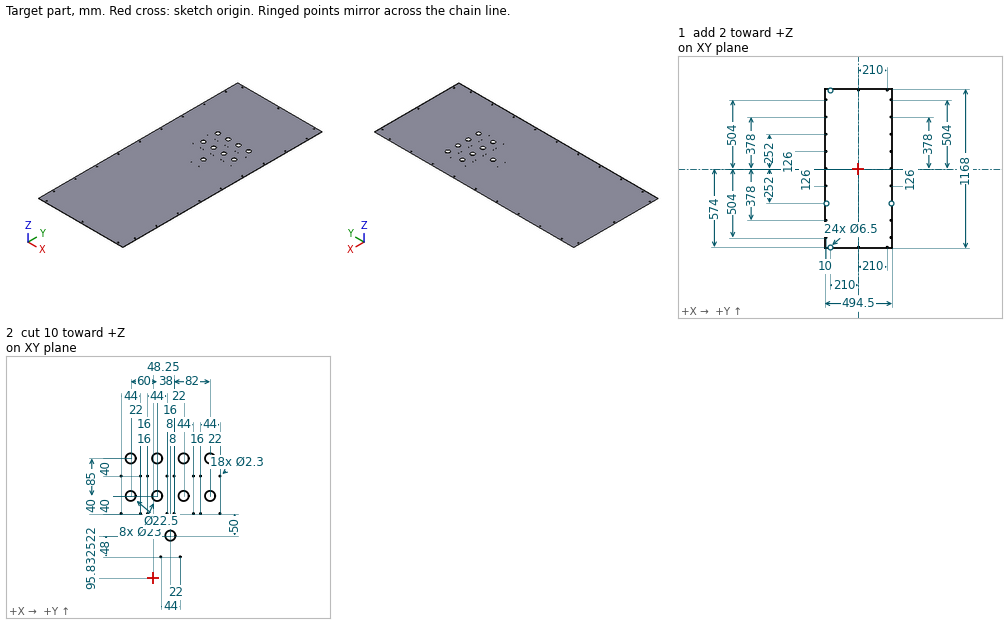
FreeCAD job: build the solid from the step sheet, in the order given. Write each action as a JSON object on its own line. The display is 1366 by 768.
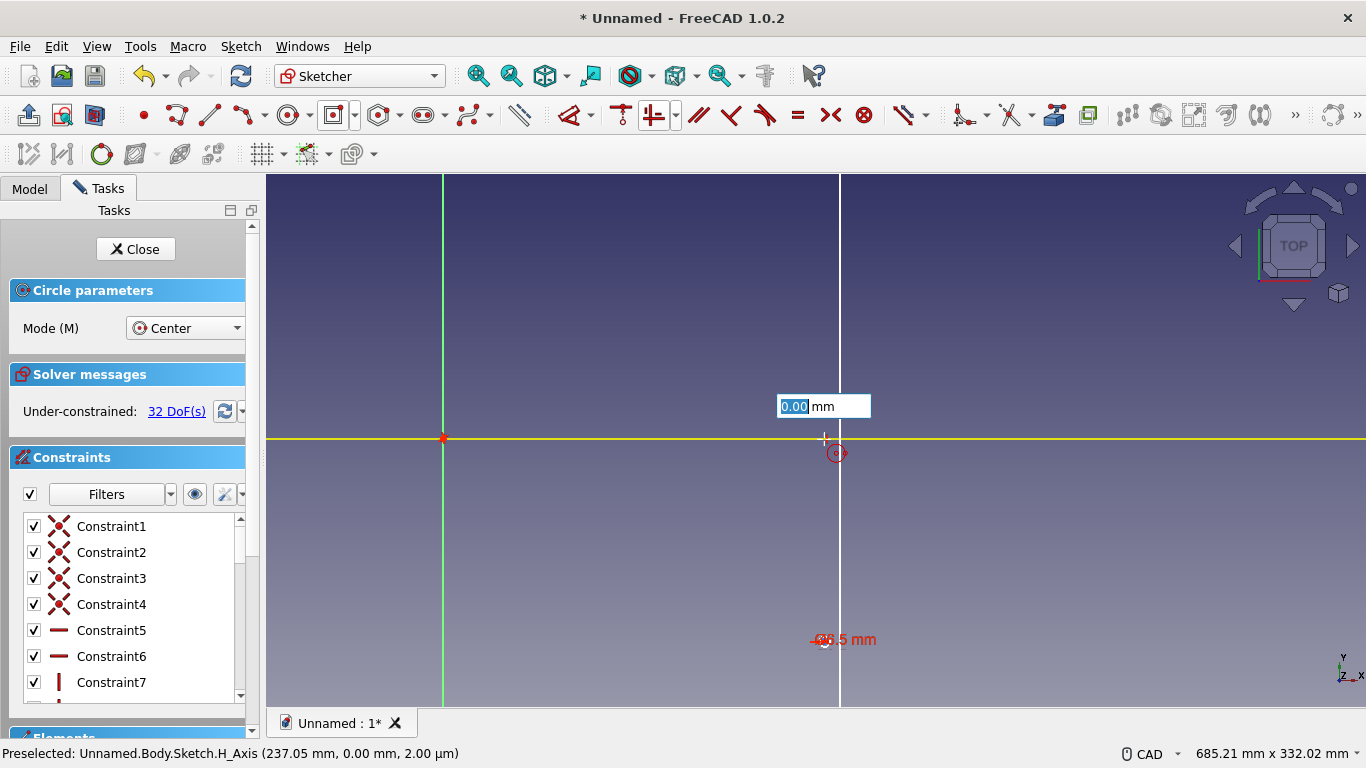
{"action": "scroll", "coordinate": [823, 443], "scroll_direction": "up", "scroll_amount": 6}
{"action": "mouse_move", "coordinate": [820, 443]}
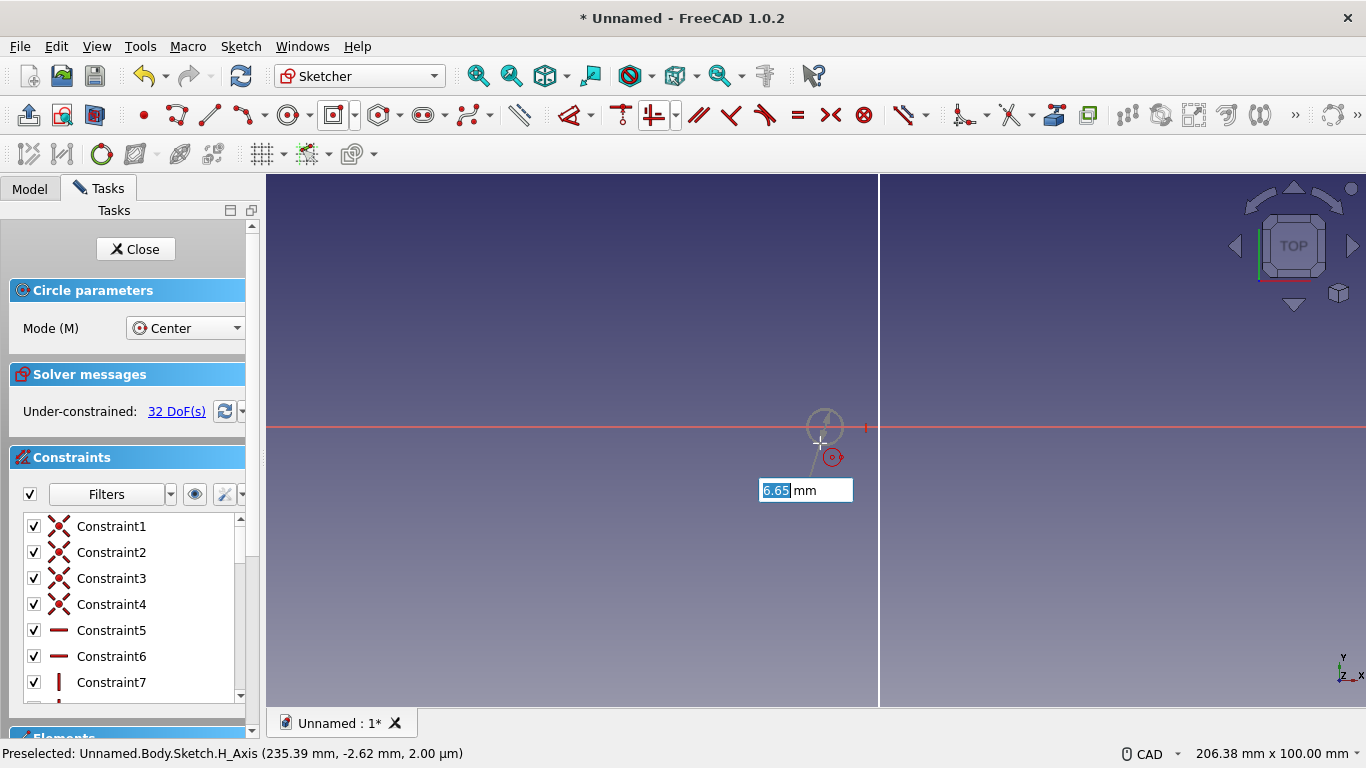
{"action": "type", "text": "6.5"}
{"action": "key", "text": "Return"}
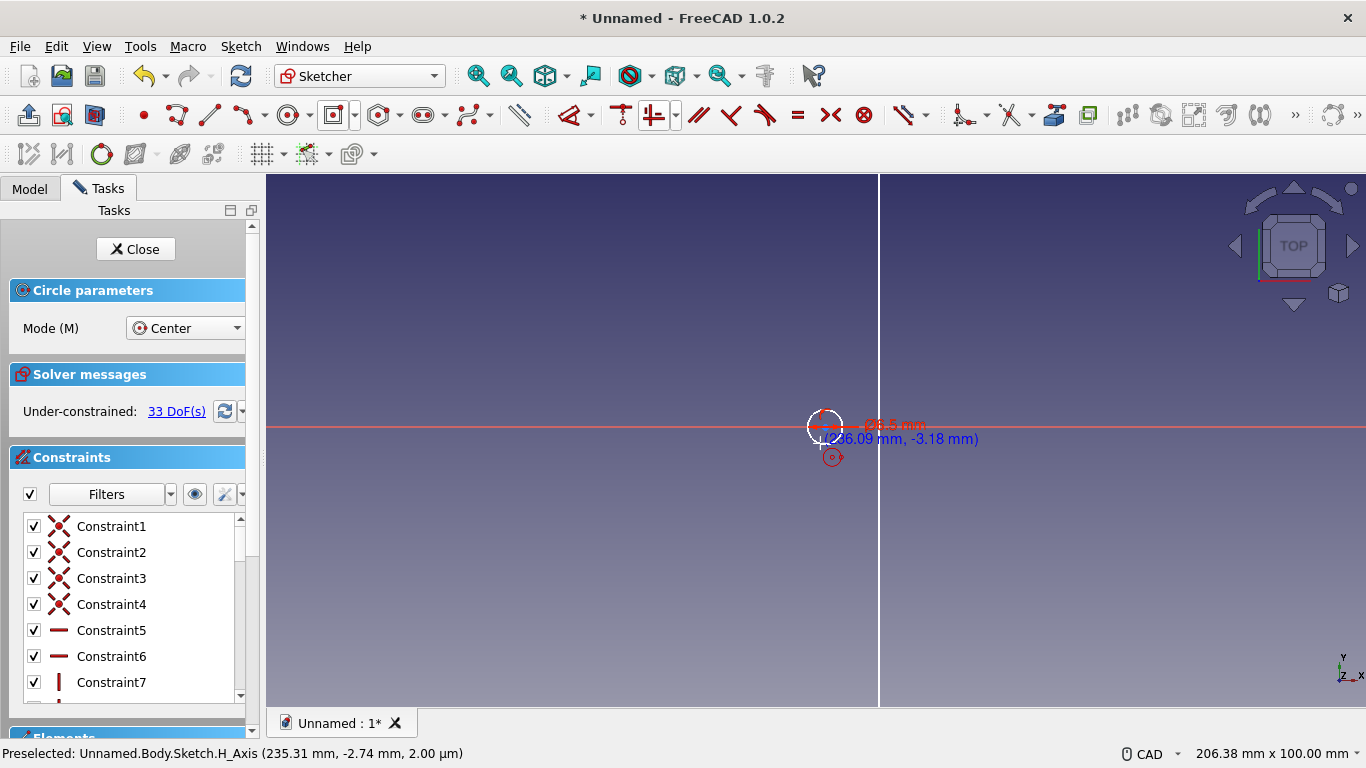
{"action": "scroll", "coordinate": [810, 441], "scroll_direction": "down", "scroll_amount": 15}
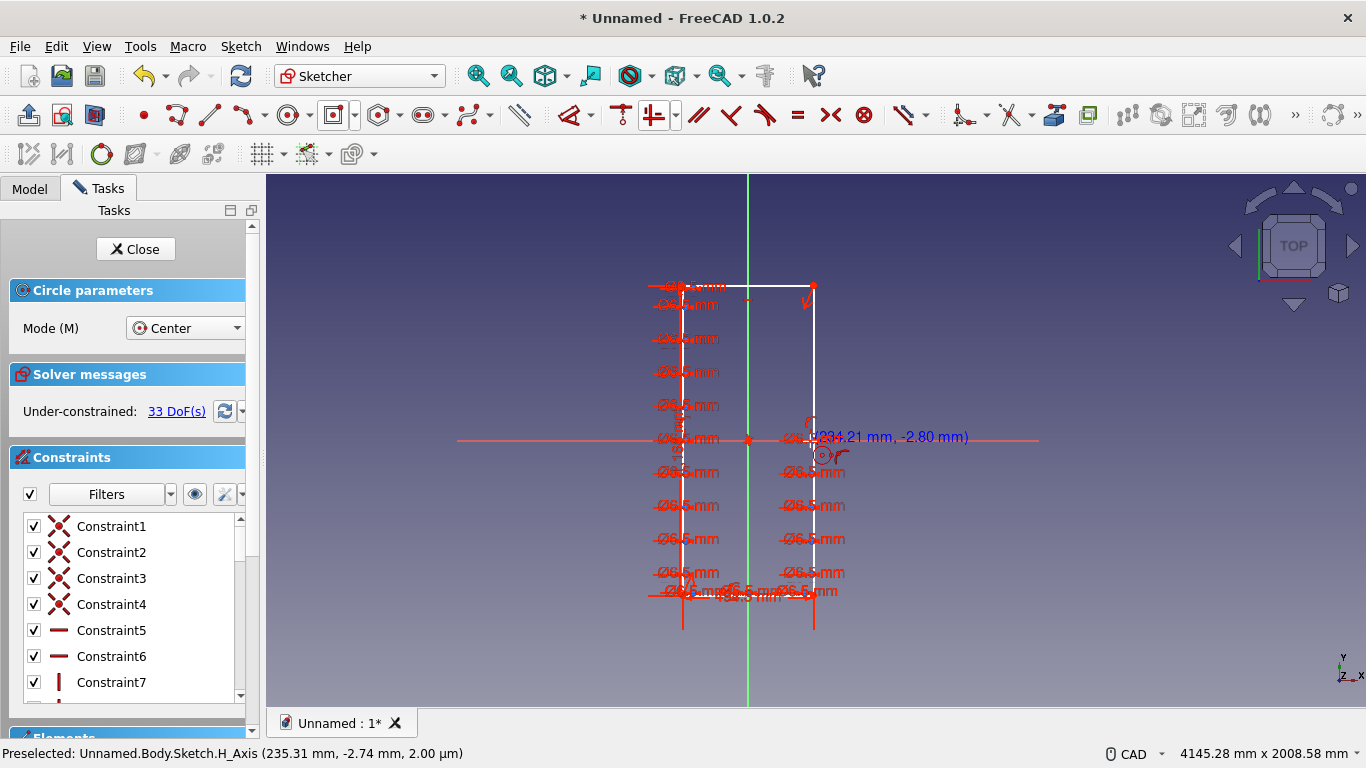
{"action": "scroll", "coordinate": [811, 407], "scroll_direction": "up", "scroll_amount": 17}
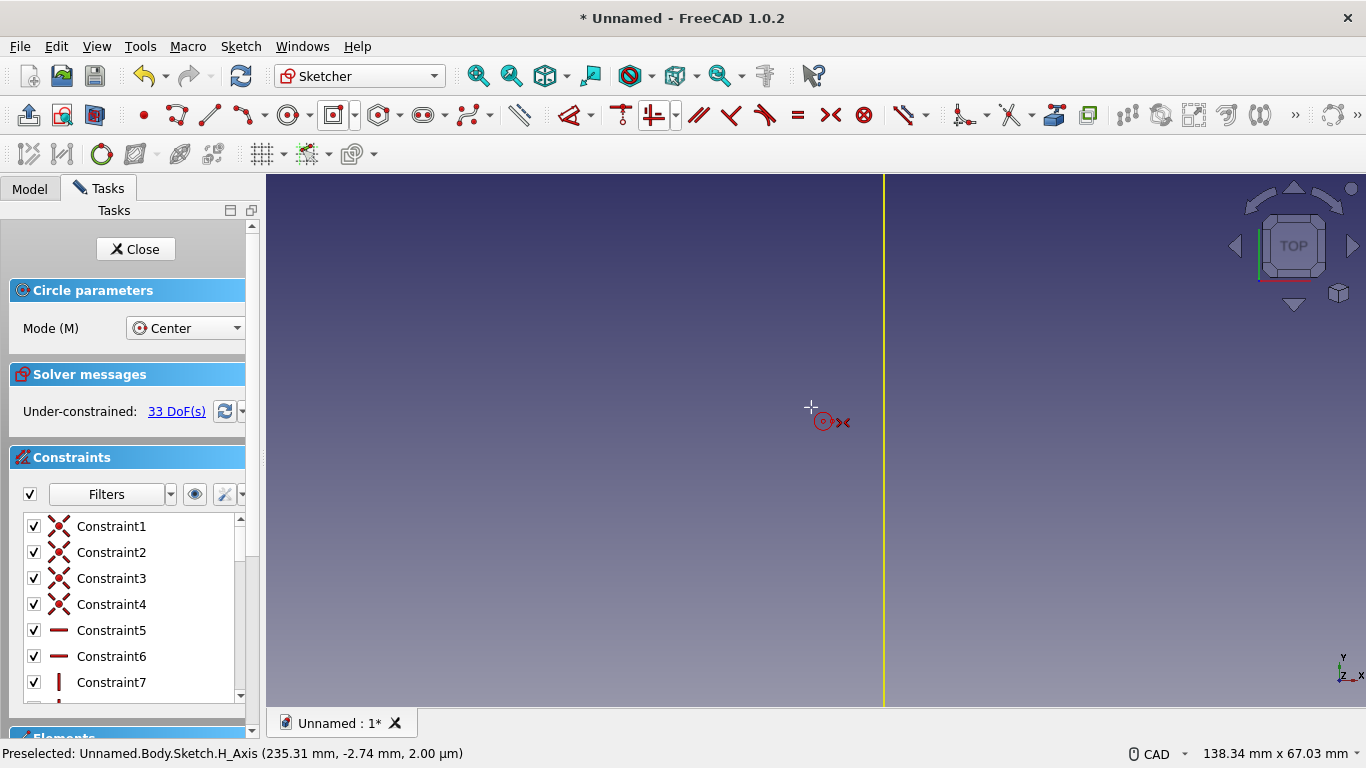
{"action": "scroll", "coordinate": [825, 399], "scroll_direction": "down", "scroll_amount": 16}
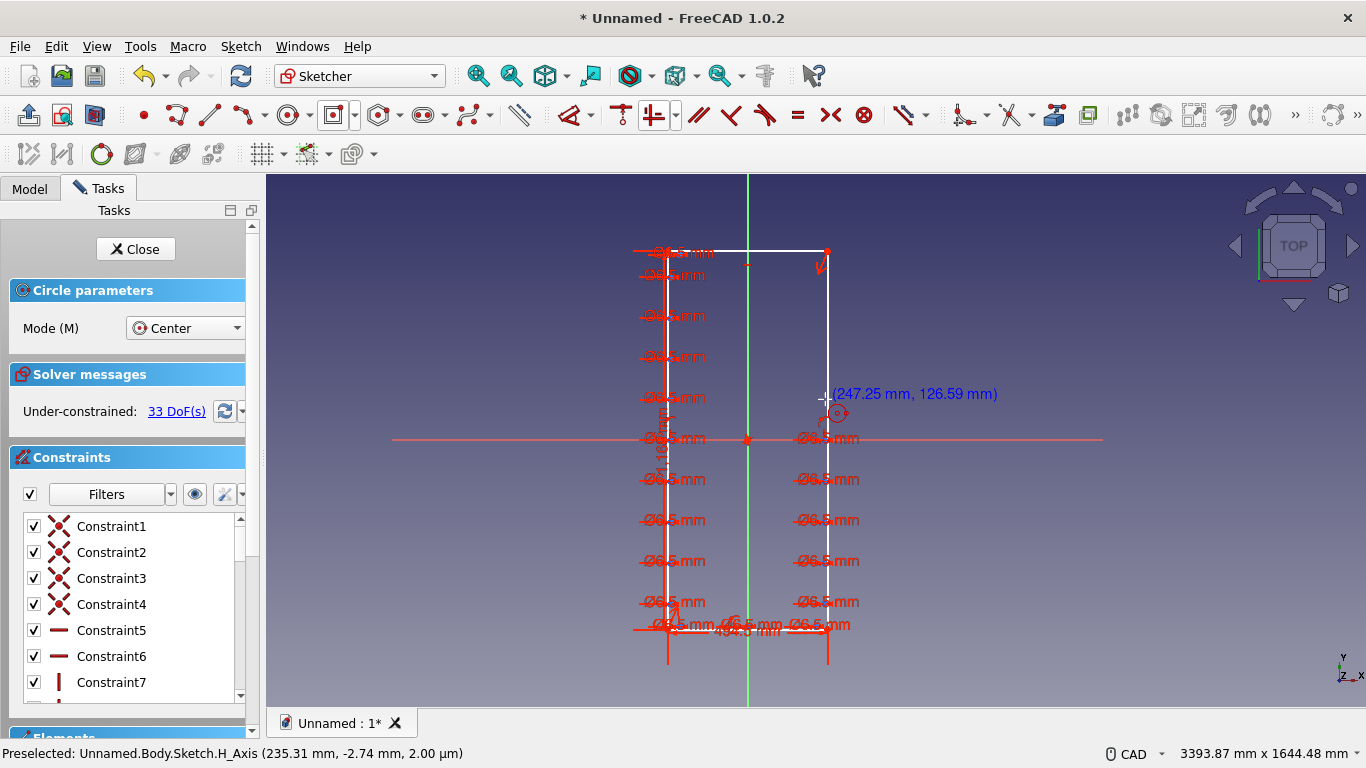
{"action": "scroll", "coordinate": [825, 400], "scroll_direction": "up", "scroll_amount": 8}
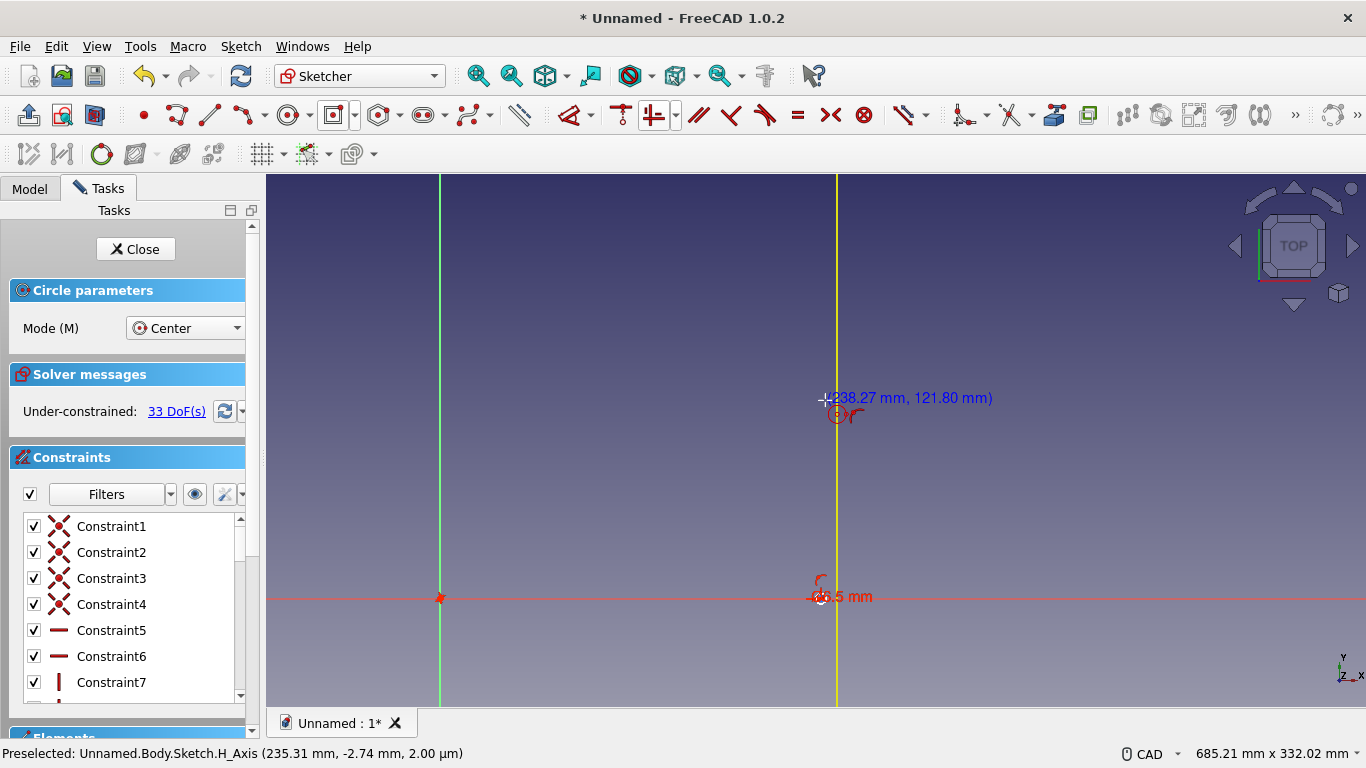
{"action": "left_click", "coordinate": [821, 397]}
{"action": "mouse_move", "coordinate": [818, 393]}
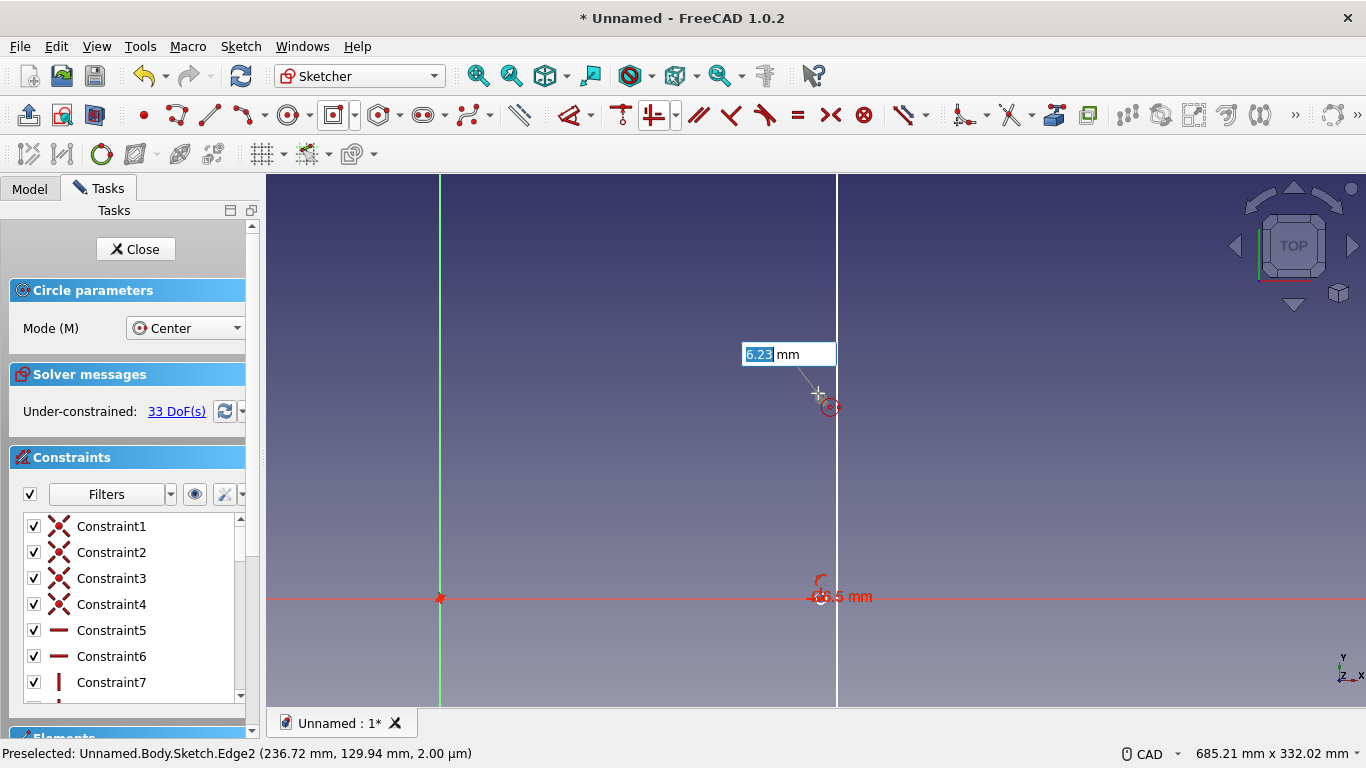
{"action": "type", "text": "6.5"}
{"action": "key", "text": "Return"}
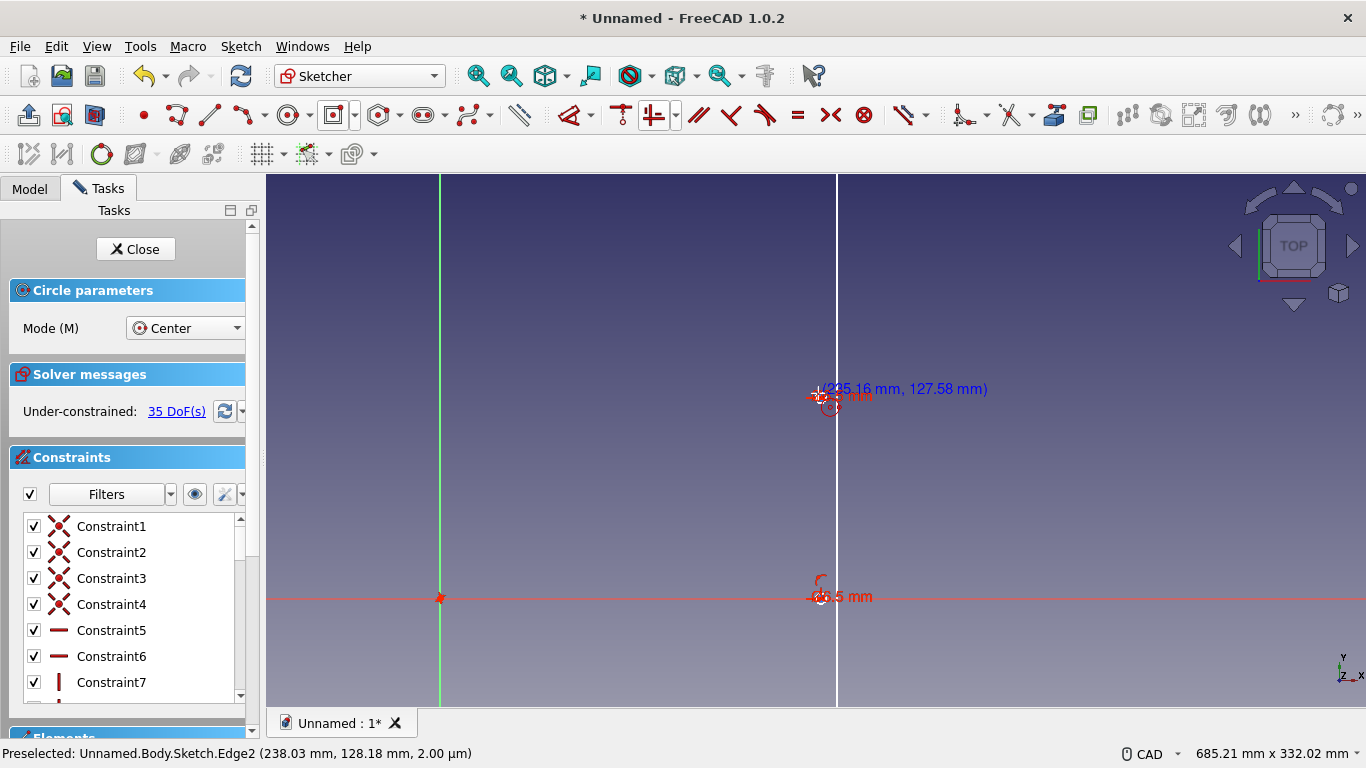
{"action": "scroll", "coordinate": [808, 409], "scroll_direction": "down", "scroll_amount": 9}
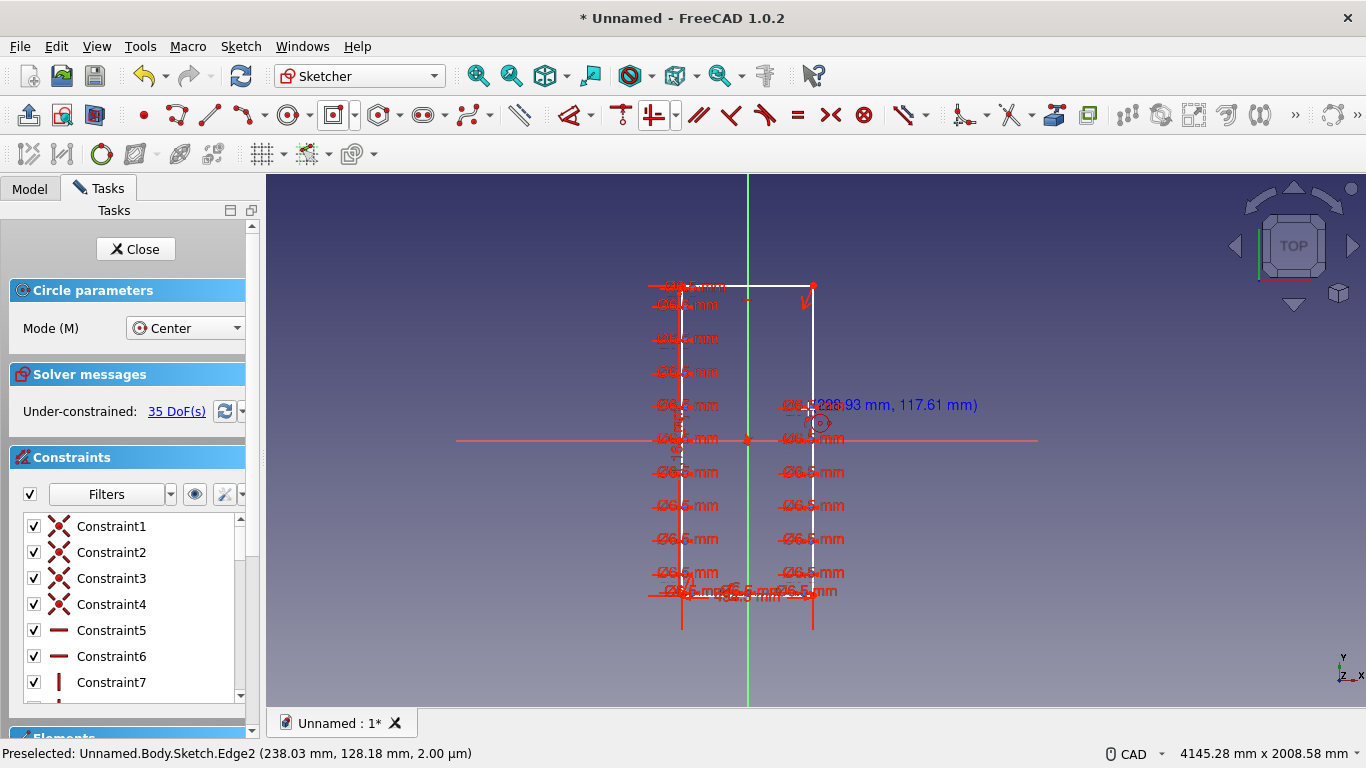
{"action": "scroll", "coordinate": [811, 374], "scroll_direction": "up", "scroll_amount": 17}